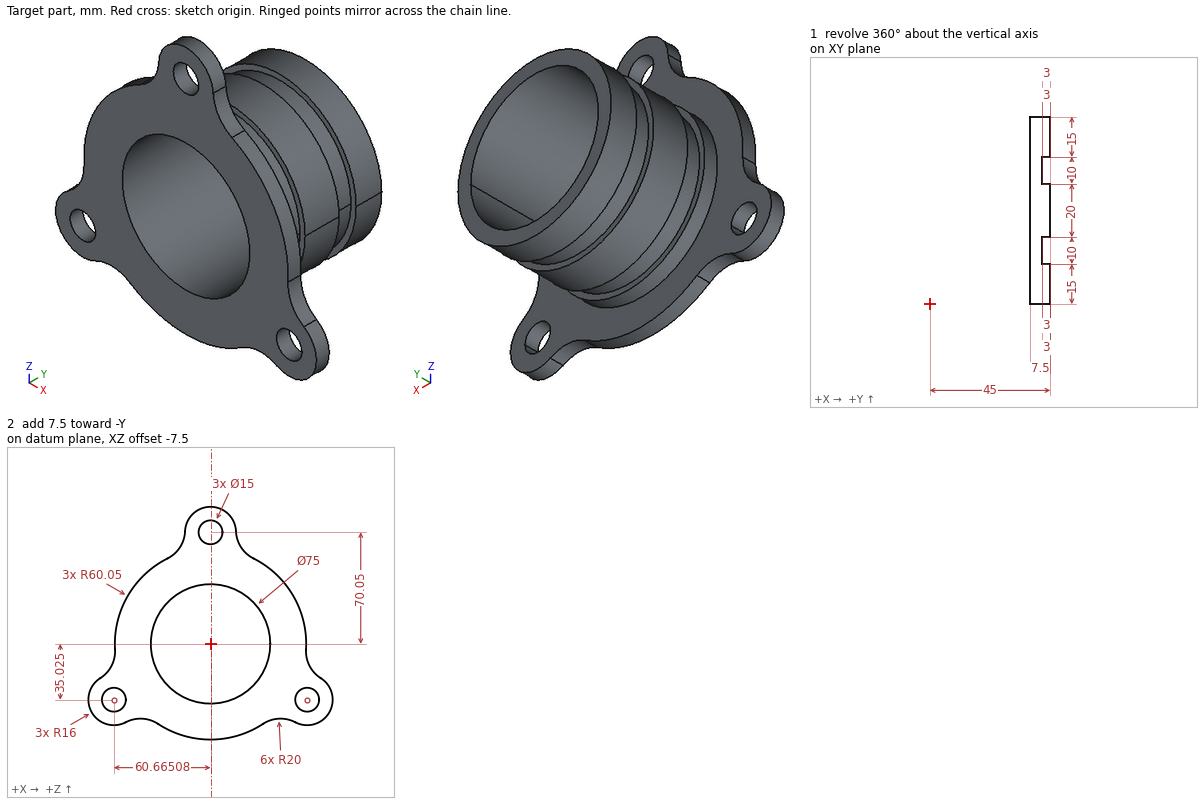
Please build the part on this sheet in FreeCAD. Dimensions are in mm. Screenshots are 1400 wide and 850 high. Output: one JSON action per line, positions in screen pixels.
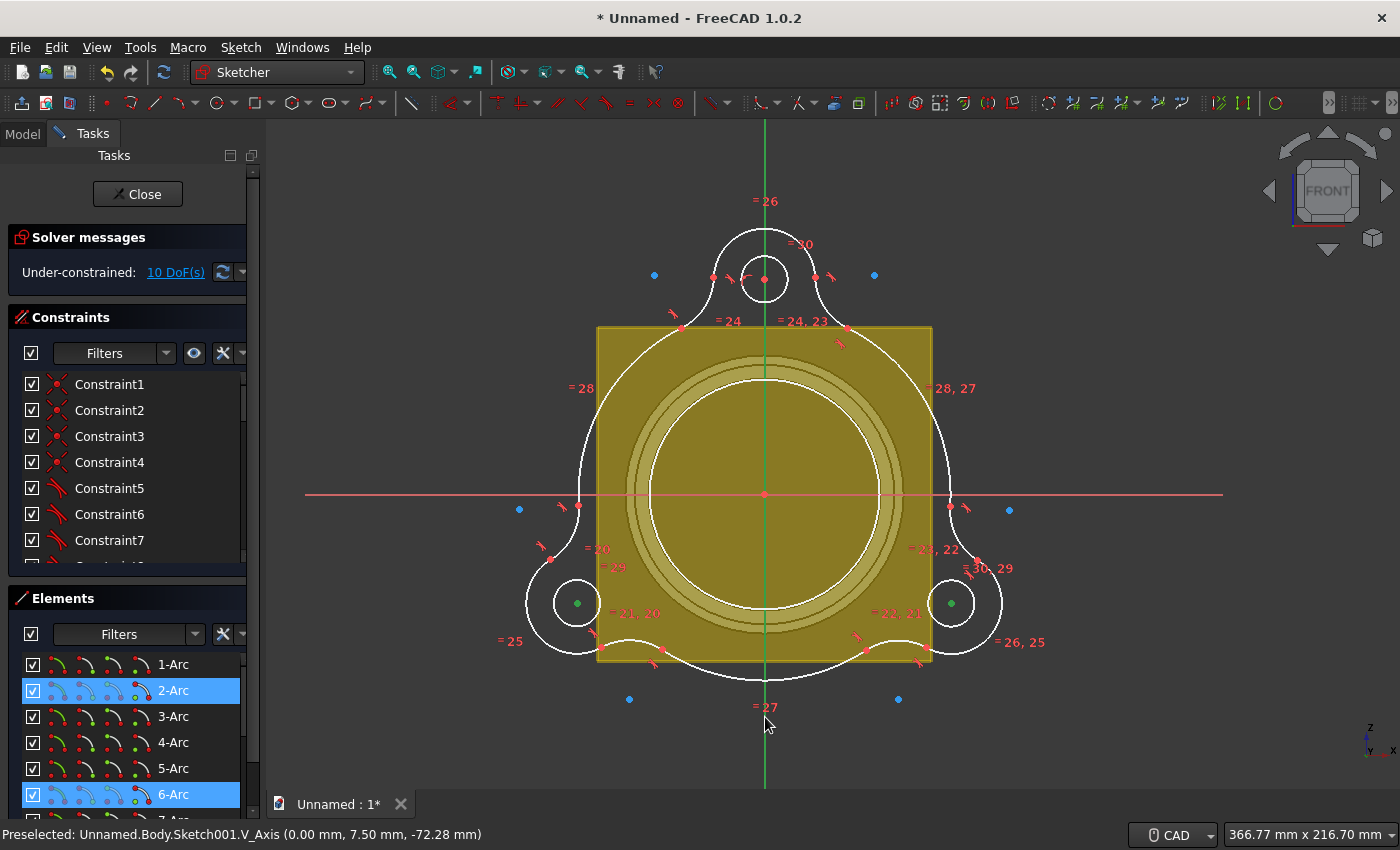
{"action": "left_click", "coordinate": [654, 104]}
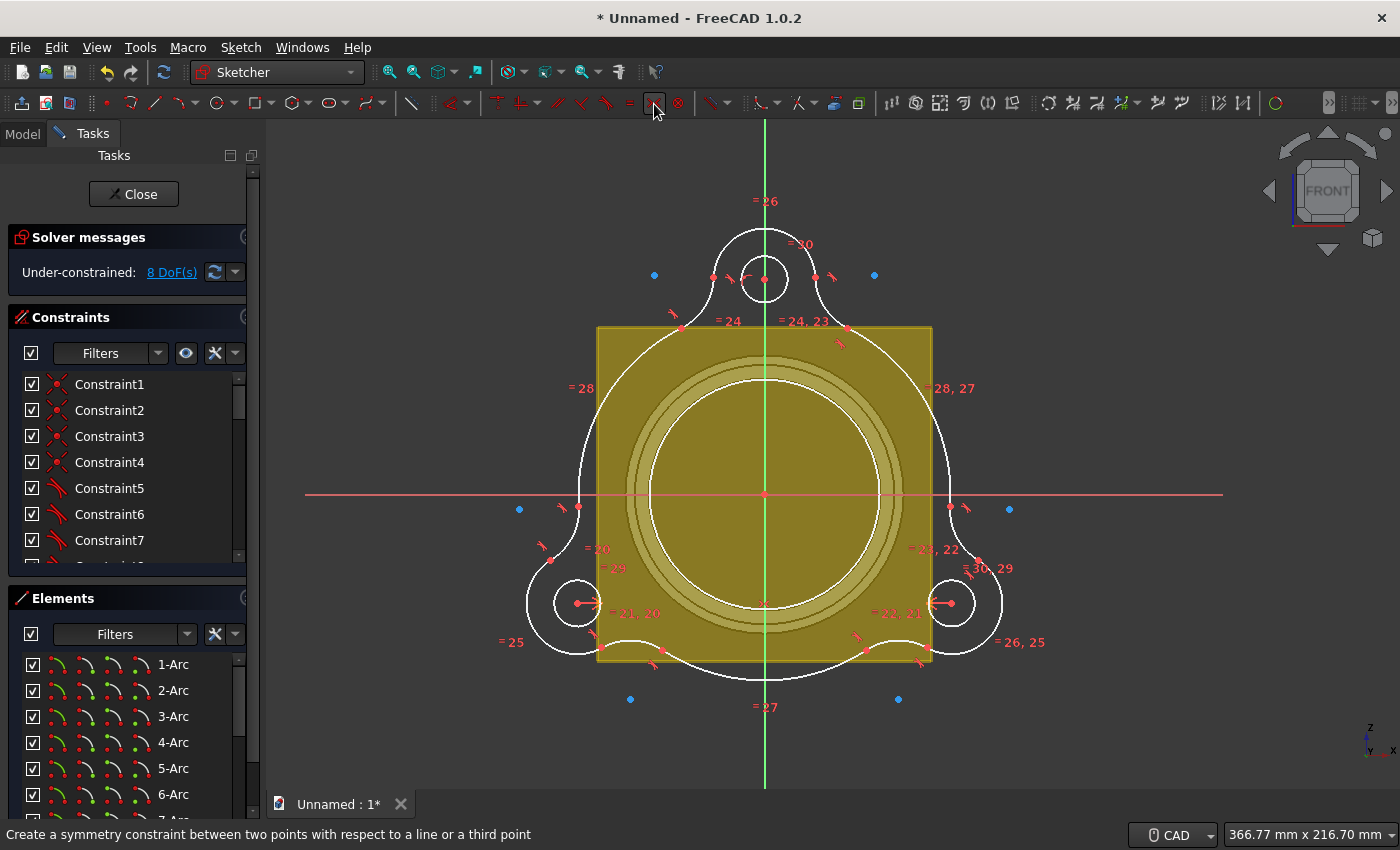
{"action": "left_click", "coordinate": [450, 104]}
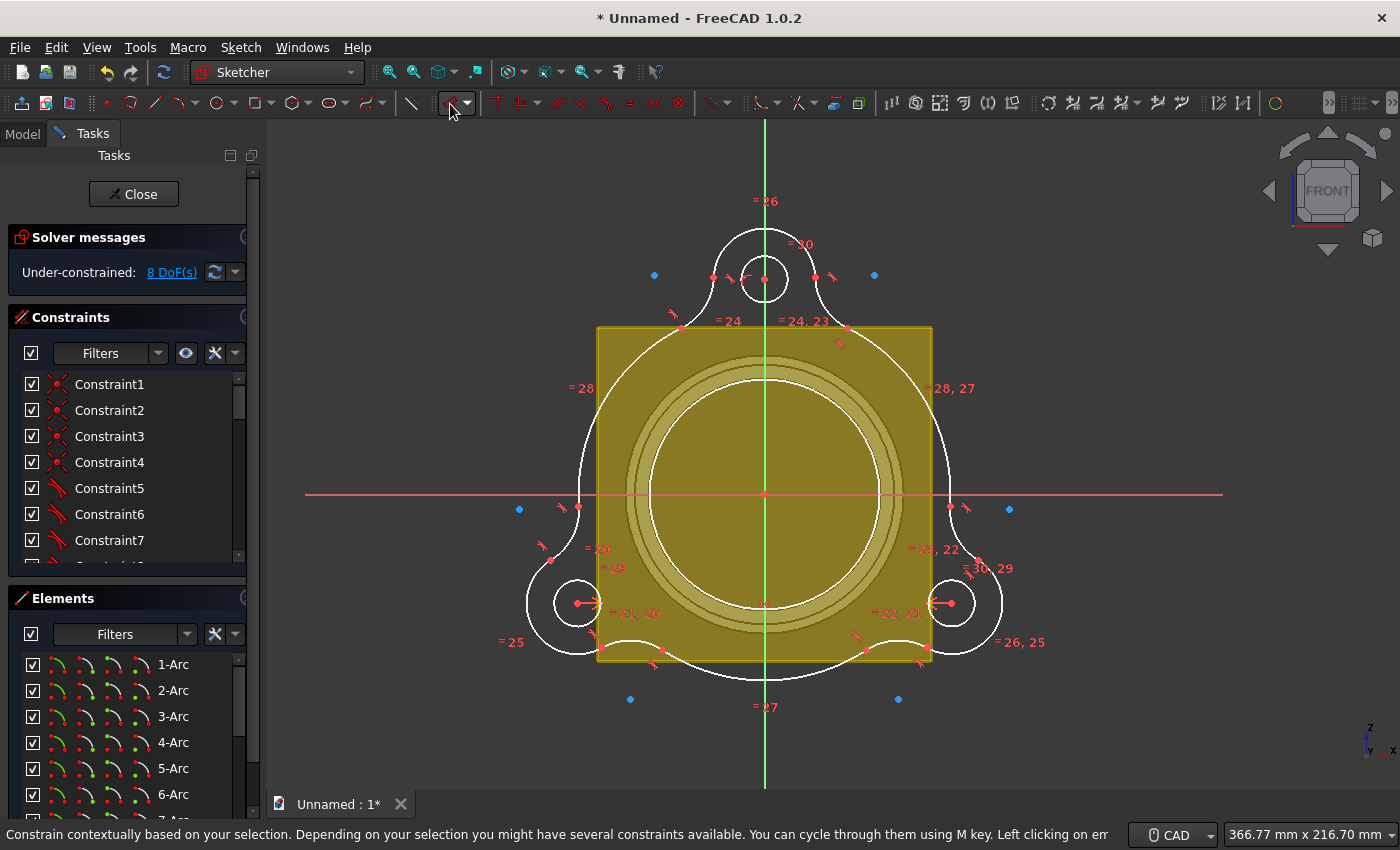
{"action": "left_click", "coordinate": [565, 548]}
{"action": "left_click", "coordinate": [589, 569]}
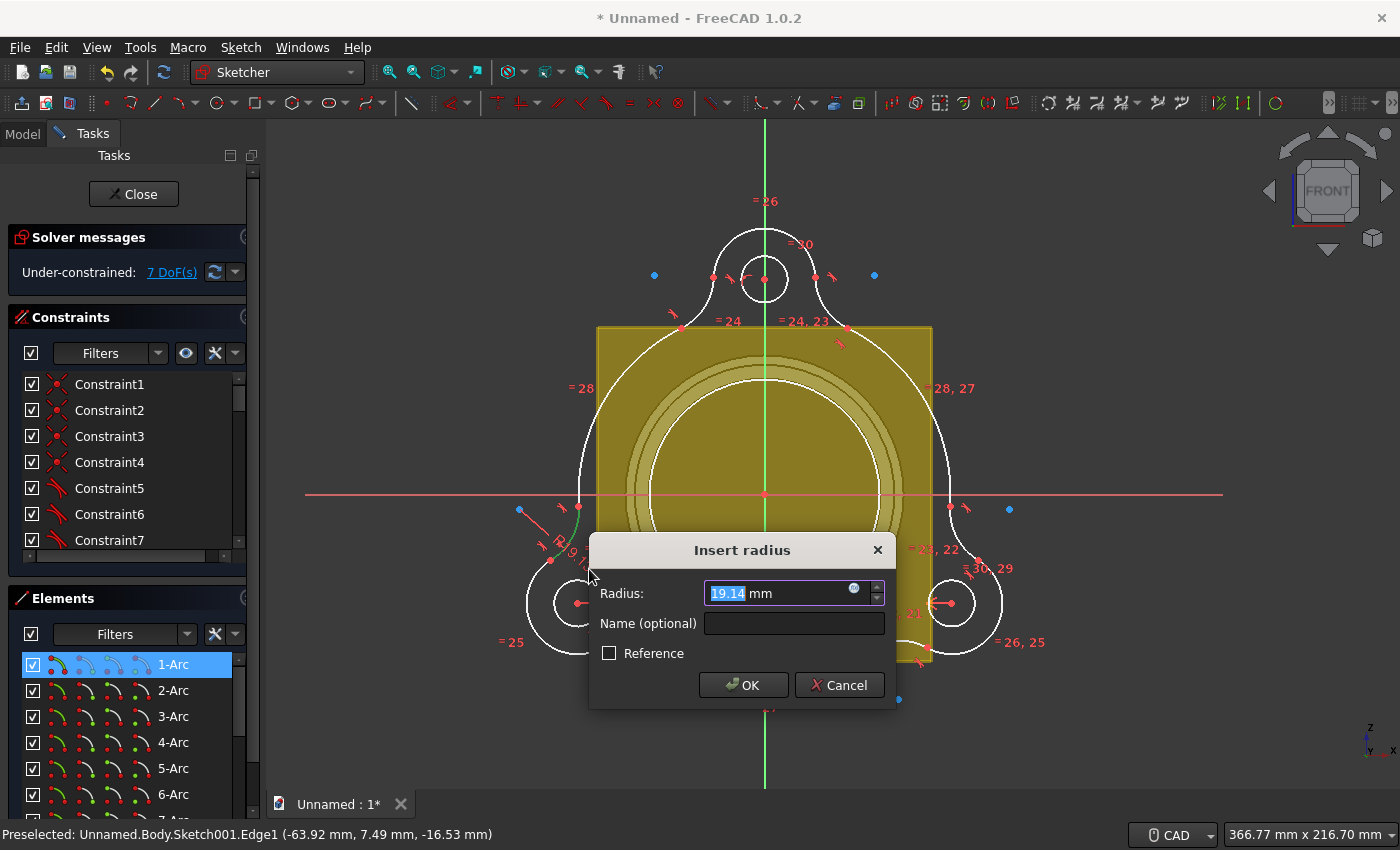
{"action": "type", "text": "20"}
{"action": "key", "text": "Return"}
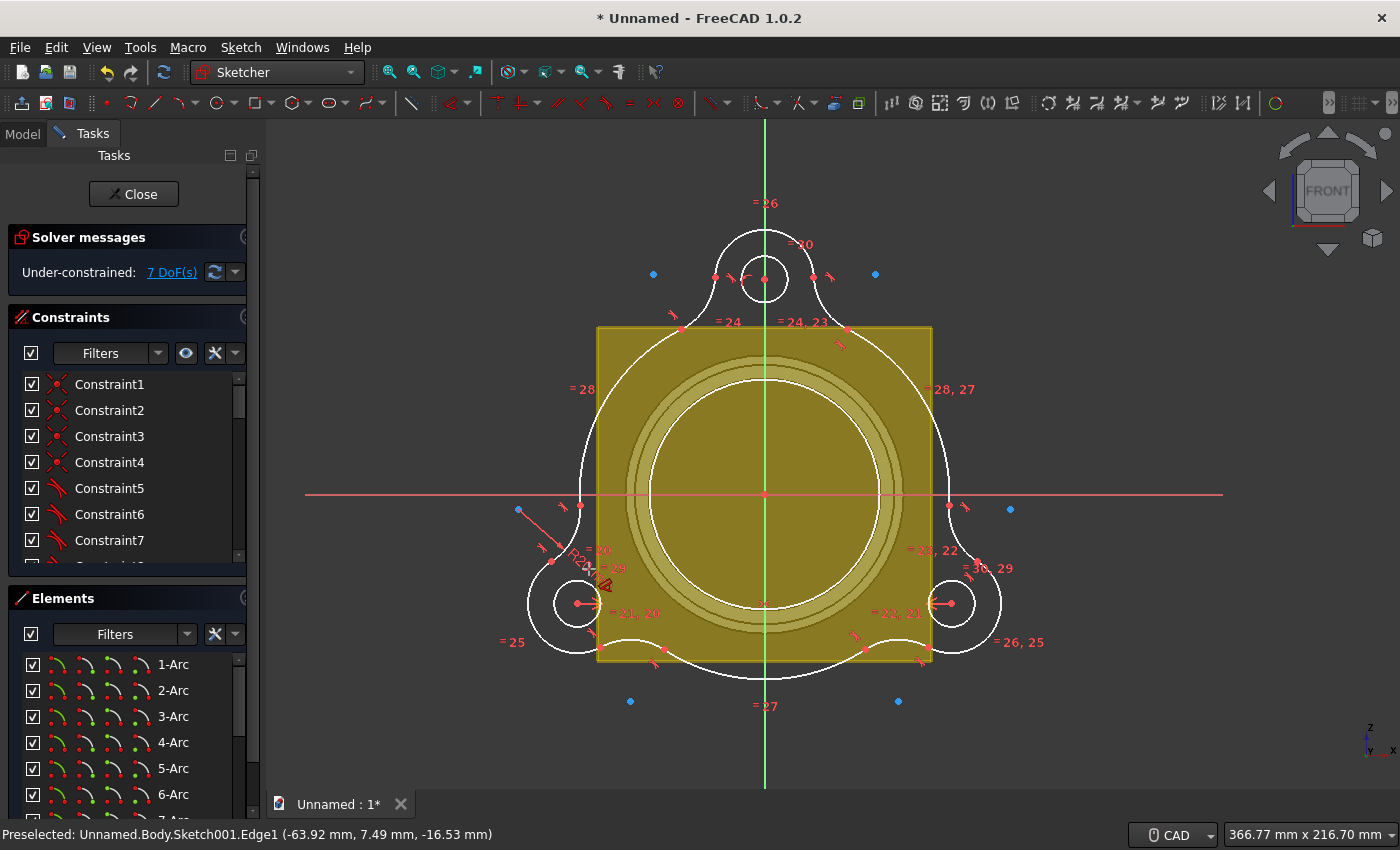
{"action": "left_click", "coordinate": [528, 599]}
{"action": "left_click", "coordinate": [496, 596]}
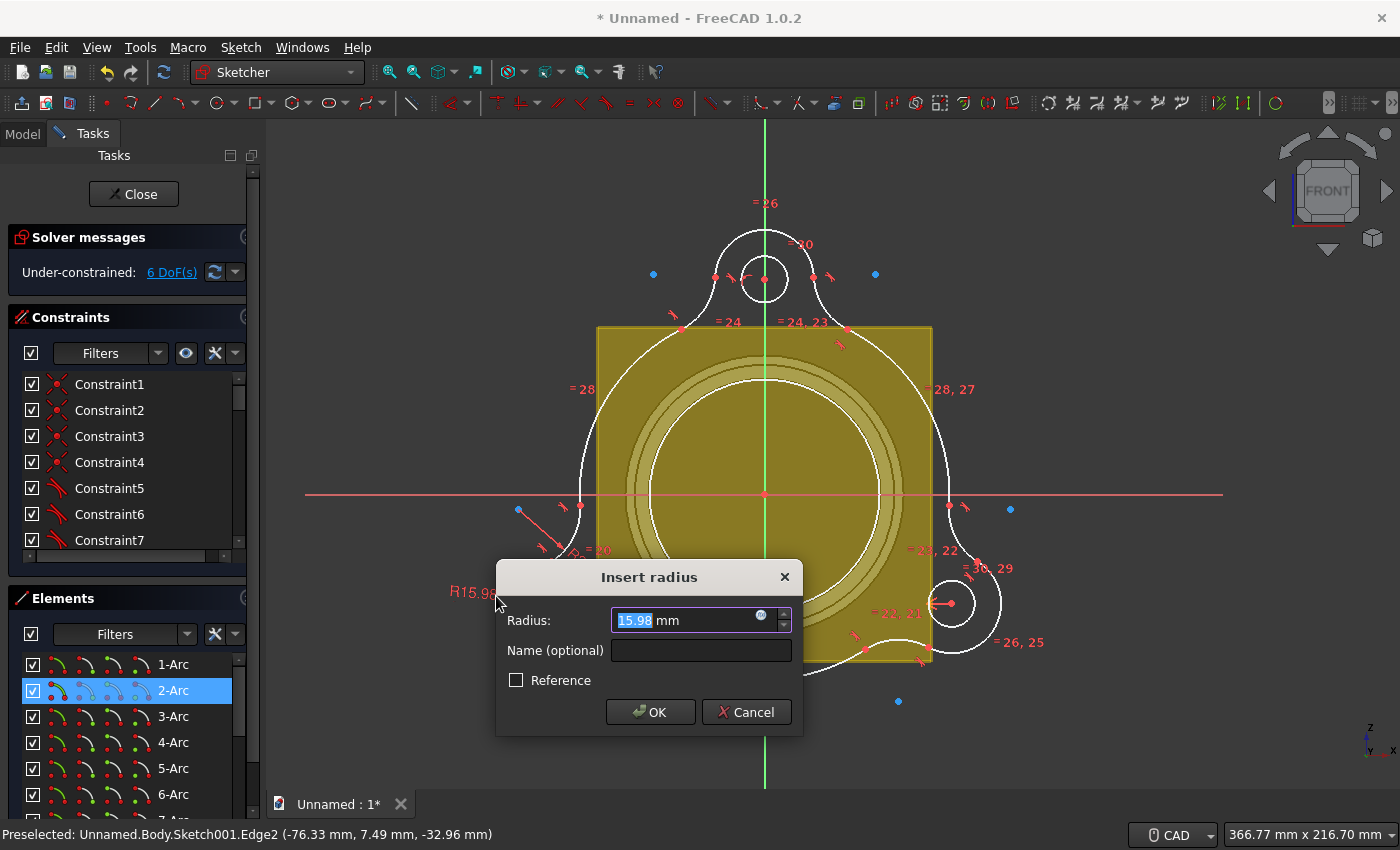
{"action": "type", "text": "16"}
{"action": "key", "text": "Return"}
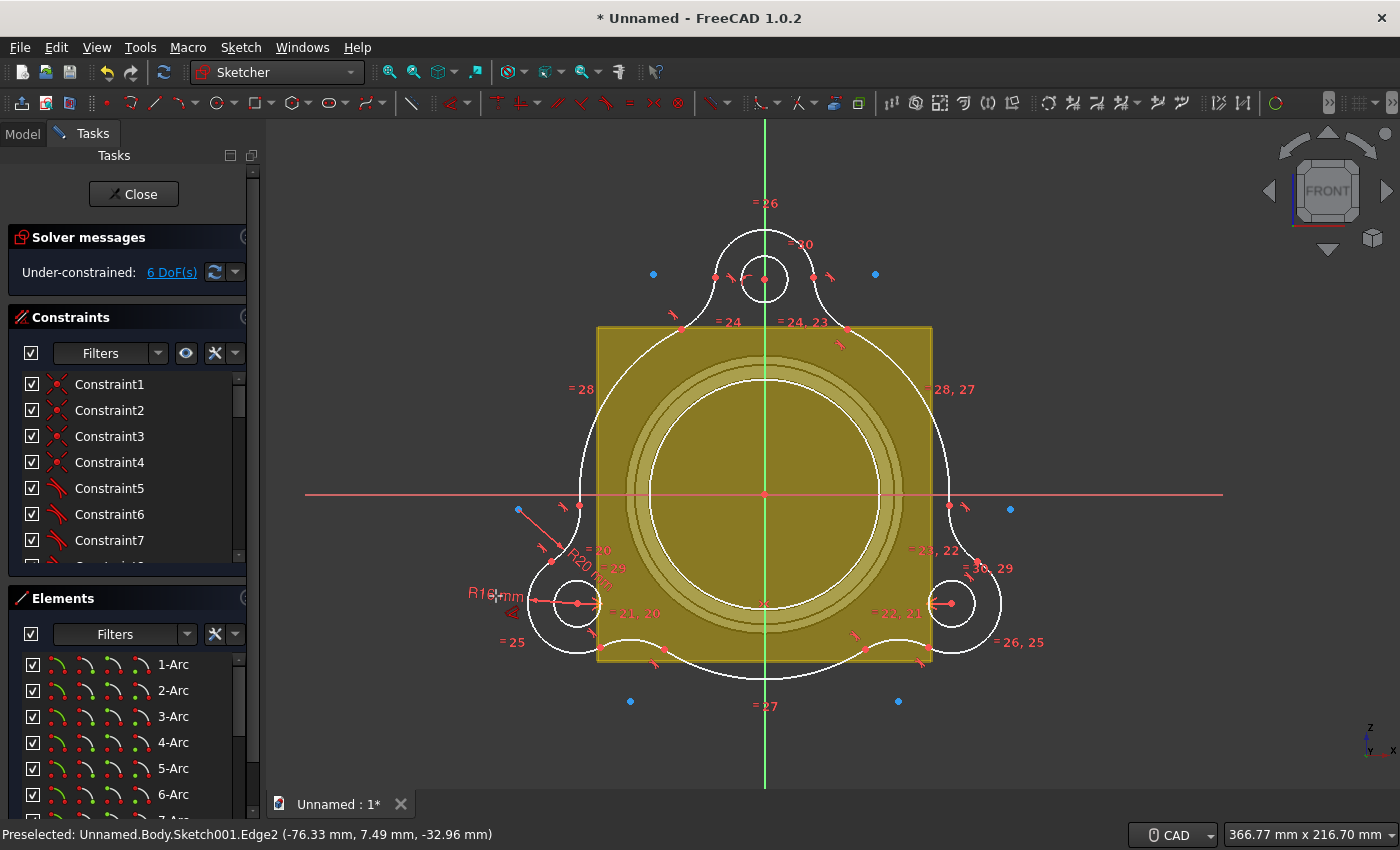
{"action": "left_click", "coordinate": [722, 675]}
{"action": "left_click", "coordinate": [715, 706]}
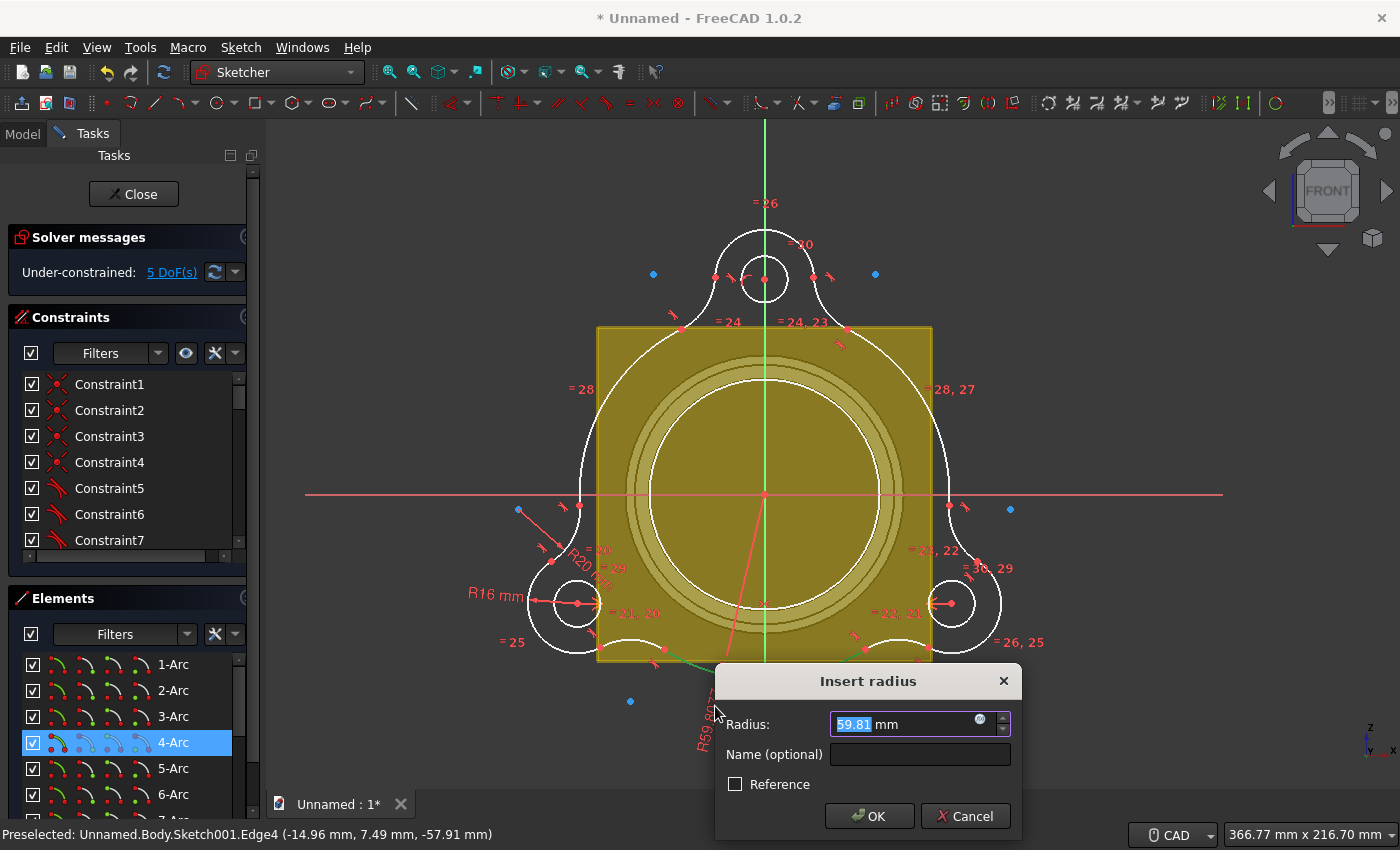
{"action": "type", "text": "60.05"}
{"action": "key", "text": "Return"}